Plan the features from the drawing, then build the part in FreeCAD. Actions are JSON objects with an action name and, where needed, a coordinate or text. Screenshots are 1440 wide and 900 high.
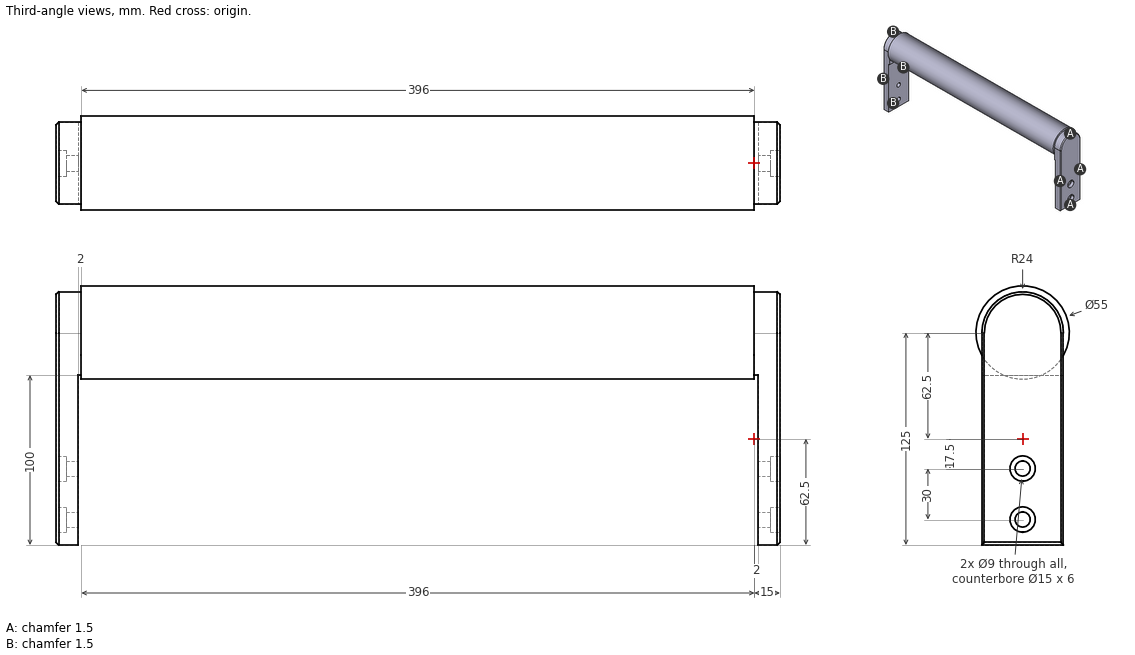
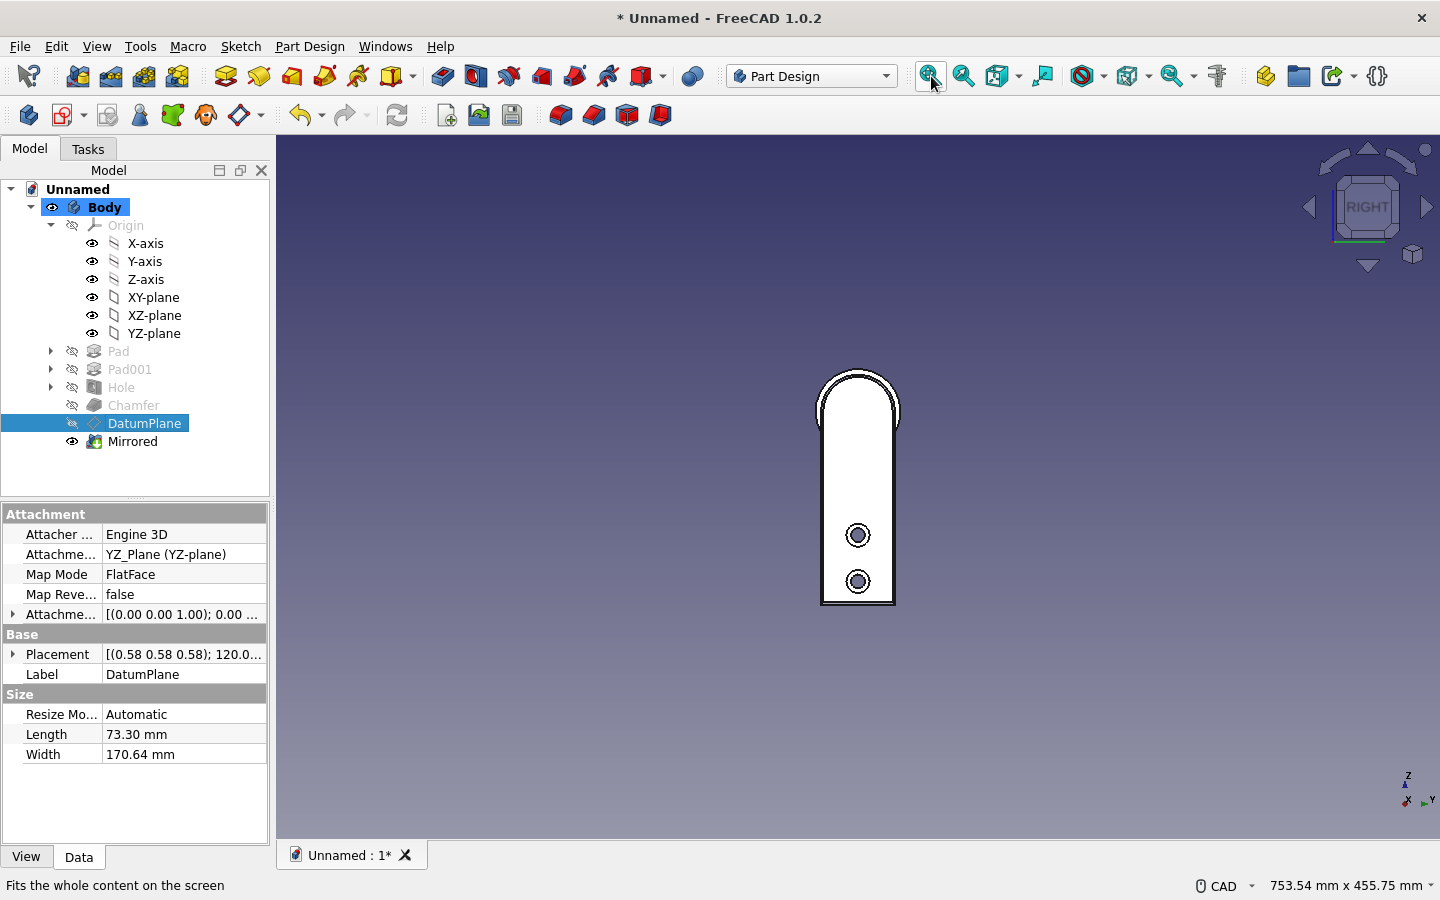
{"action": "key", "text": "0"}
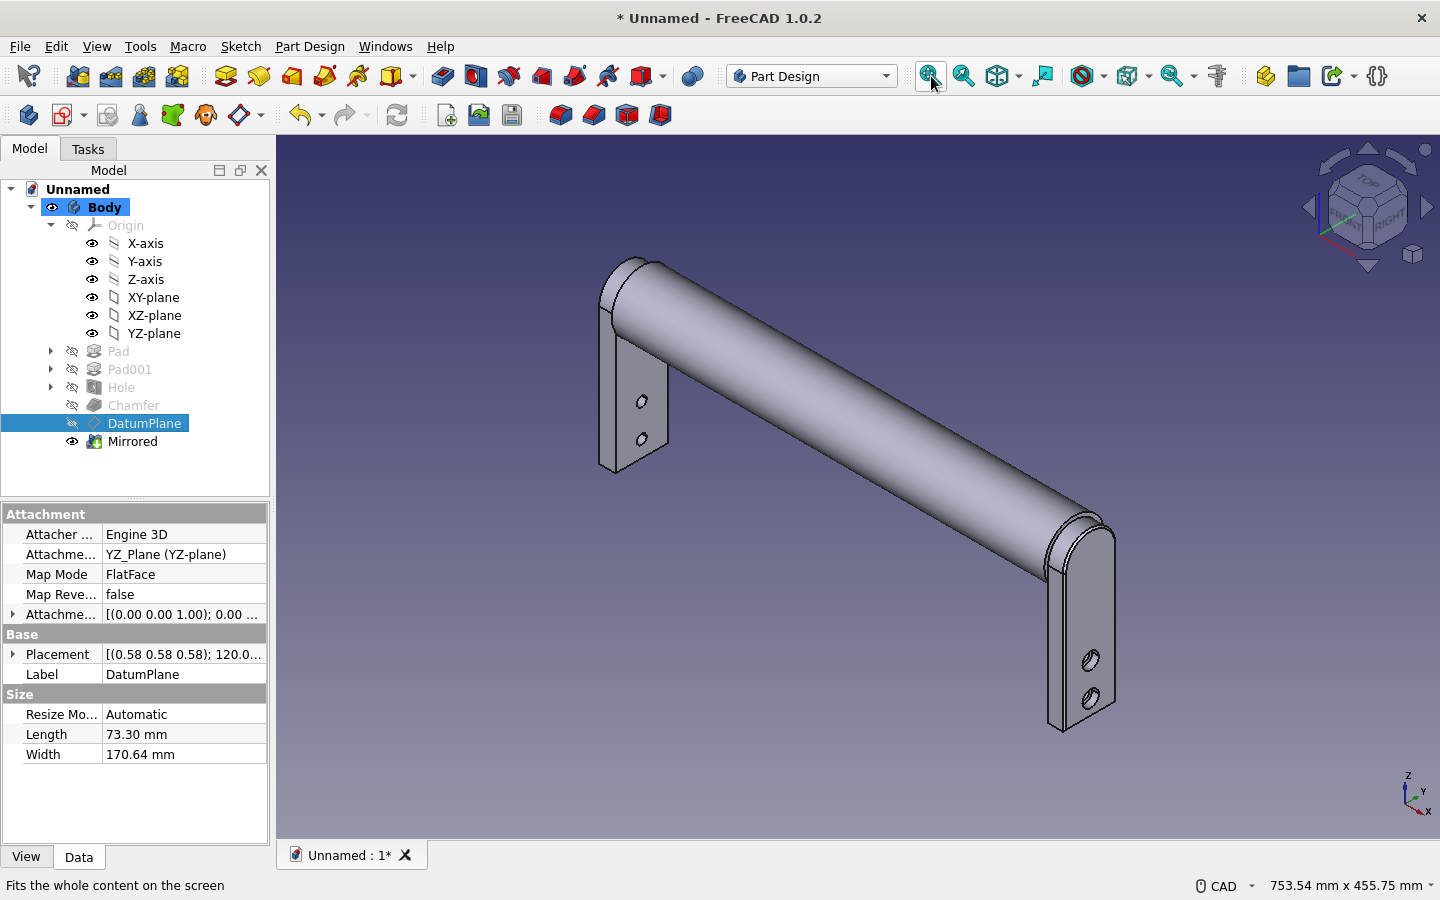
{"action": "left_click", "coordinate": [625, 260]}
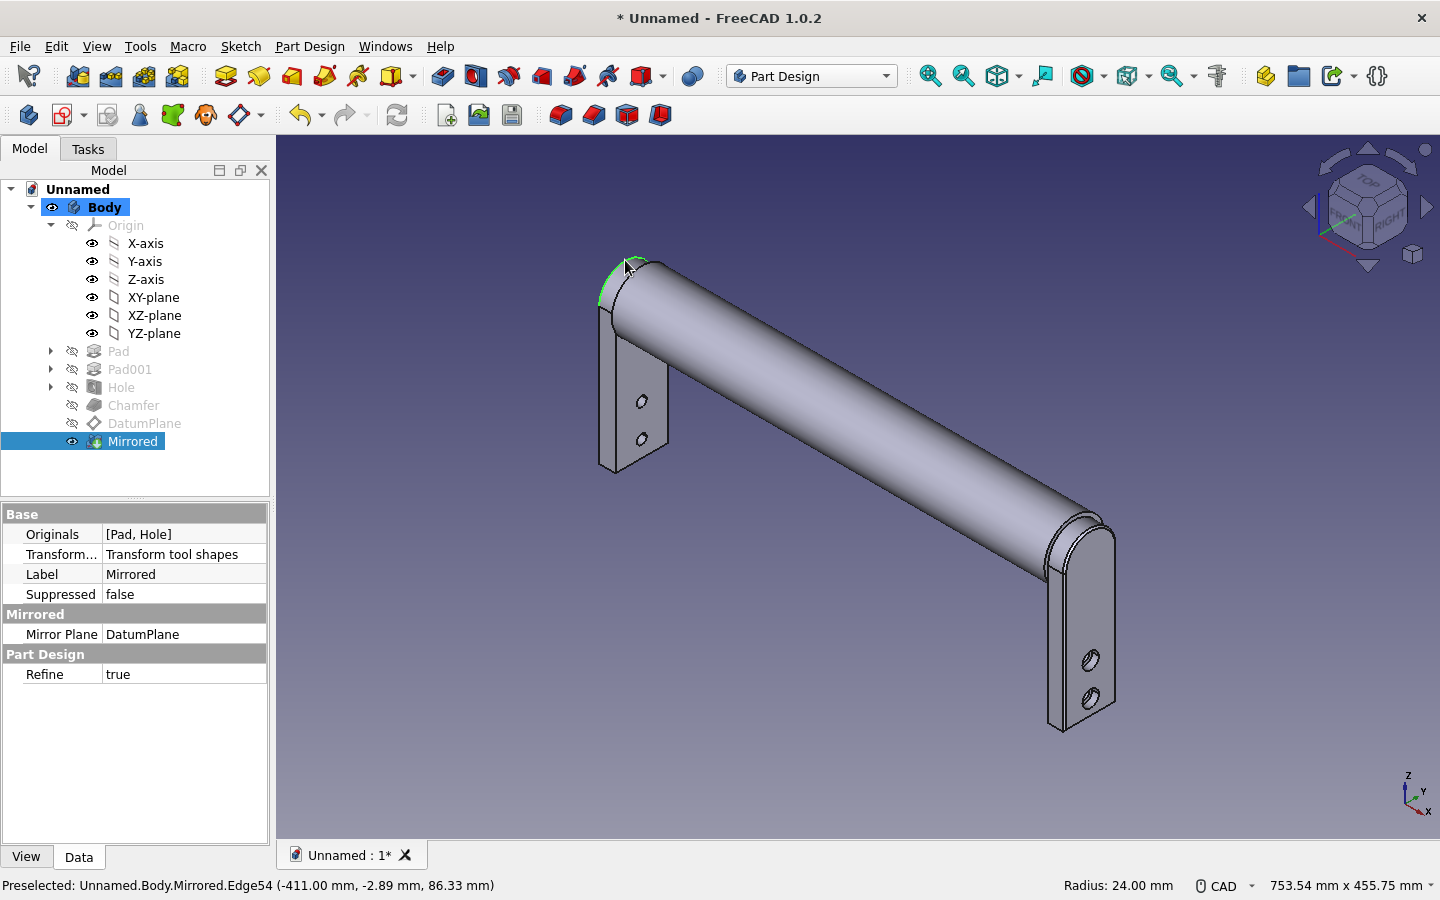
{"action": "key", "text": "2"}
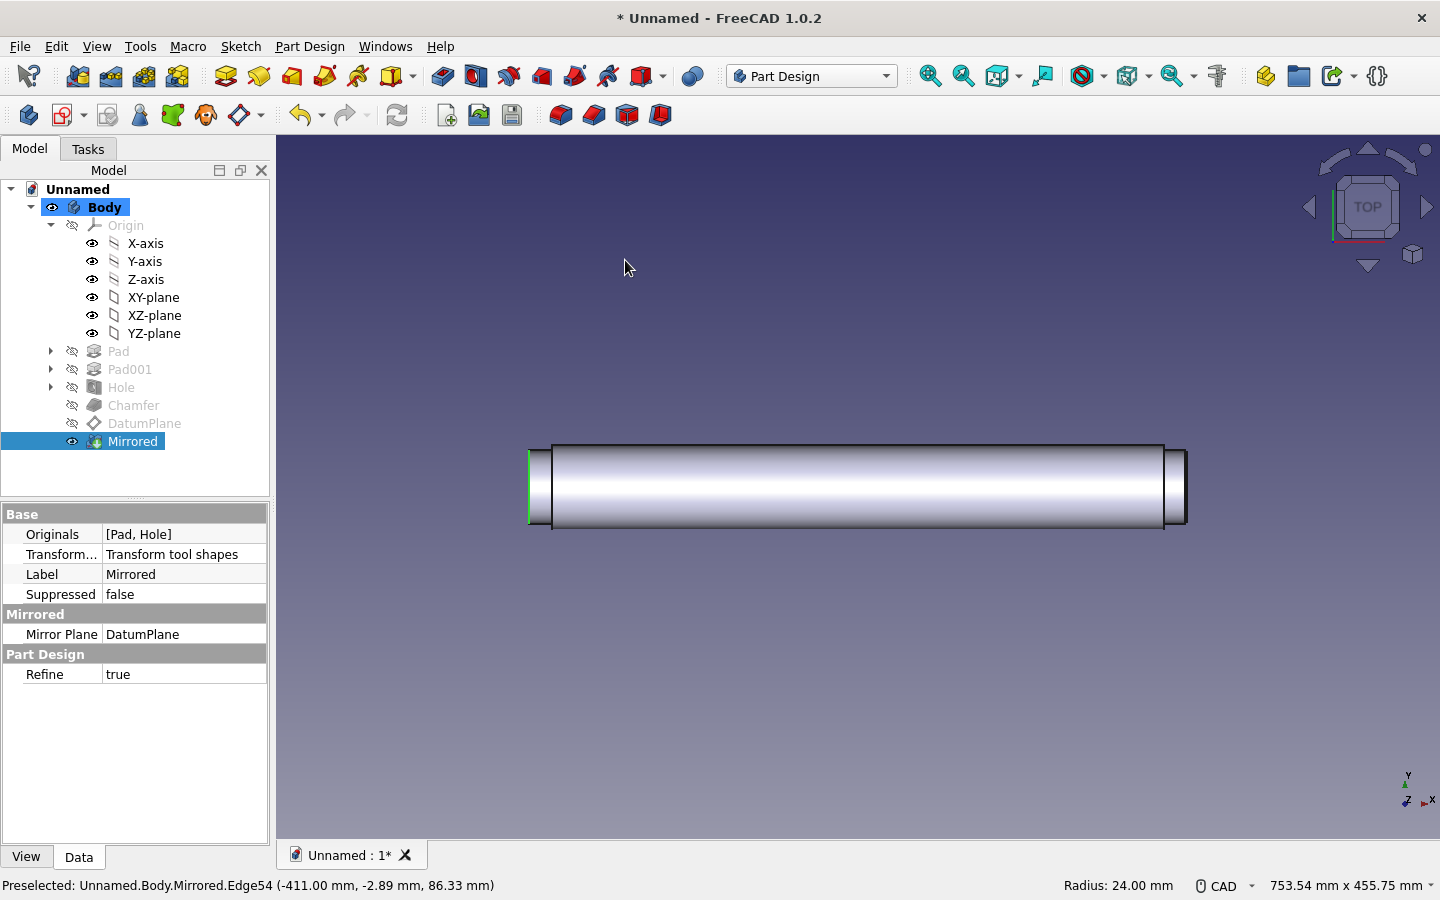
{"action": "key", "text": "1"}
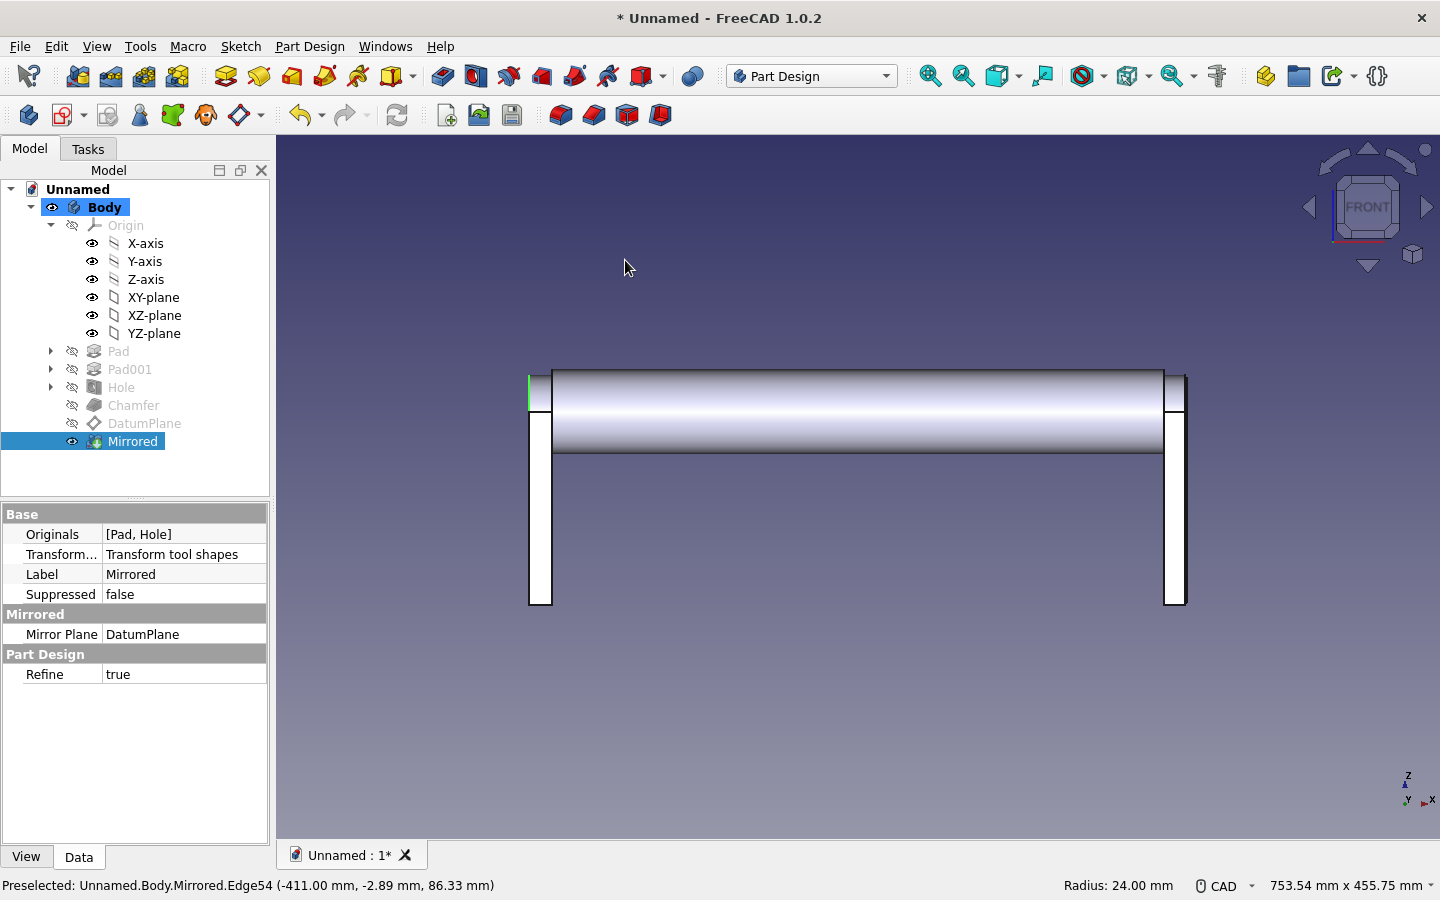
{"action": "left_click", "coordinate": [529, 507], "text": "ctrl"}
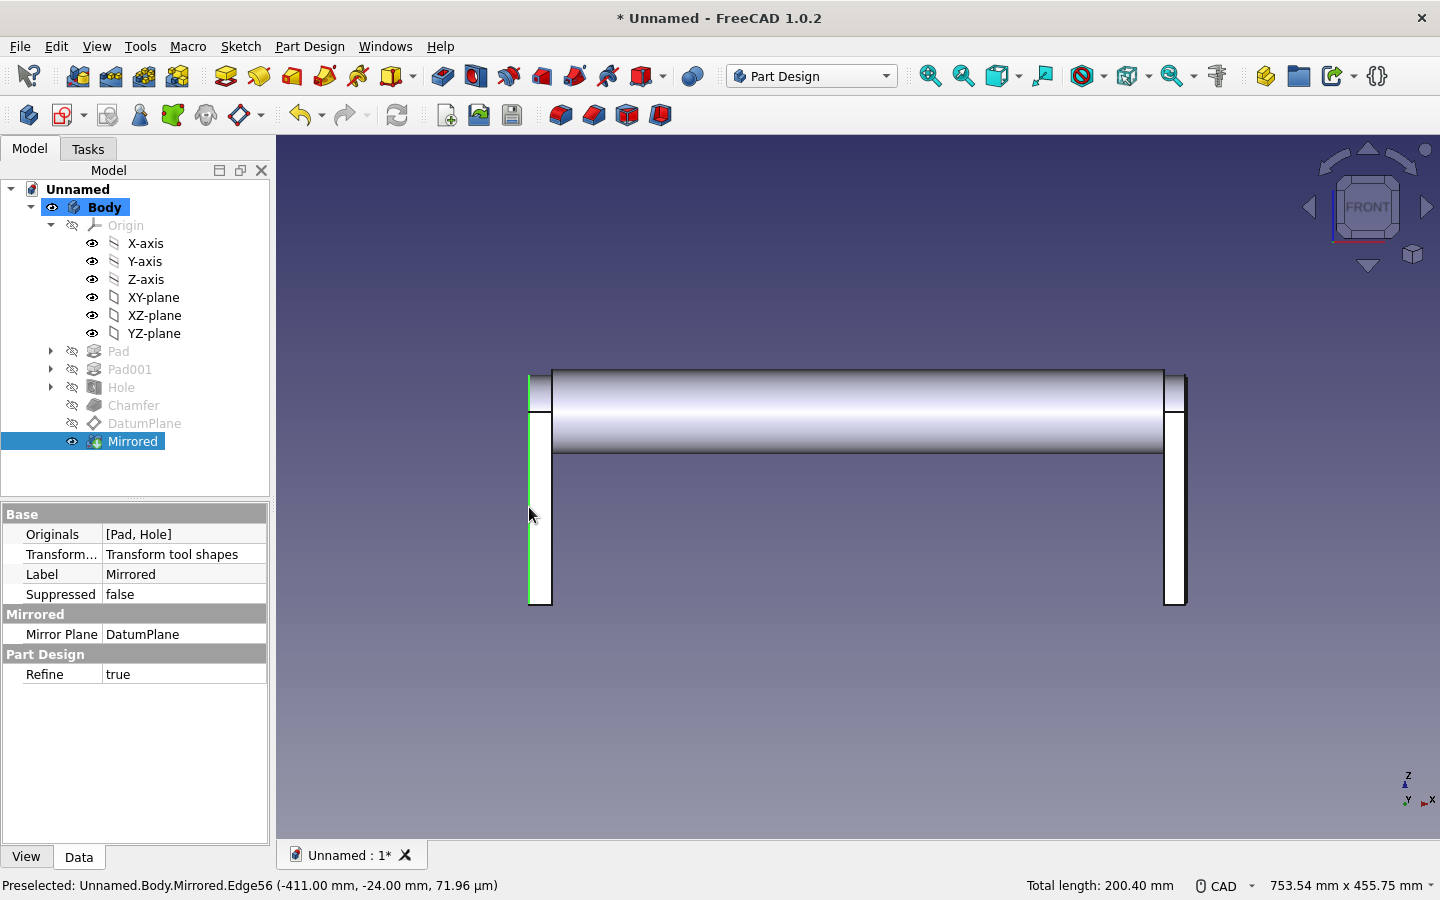
{"action": "key", "text": "3"}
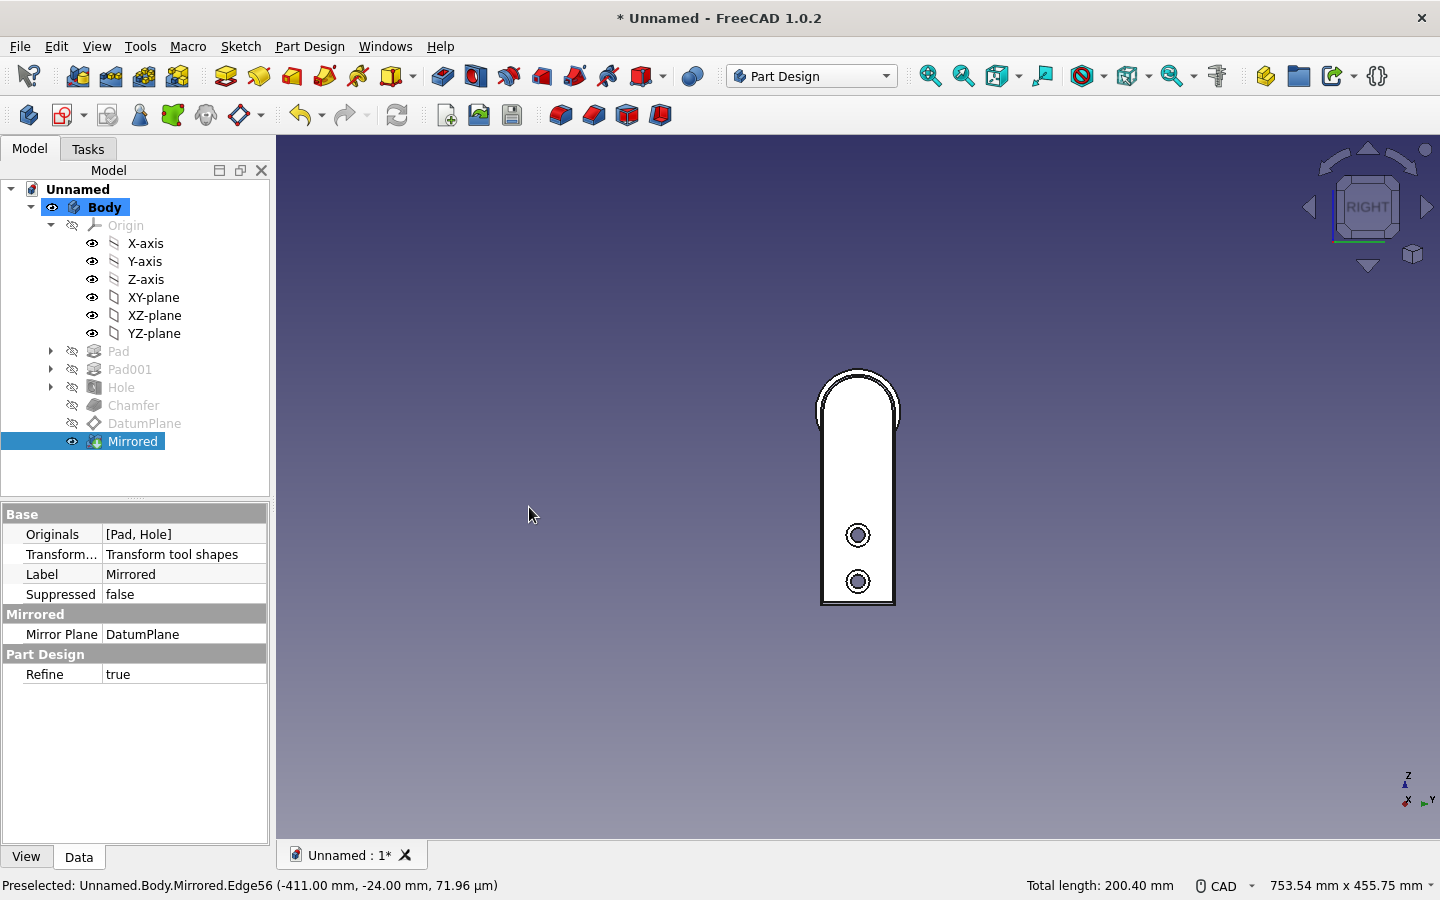
{"action": "left_click", "coordinate": [931, 76]}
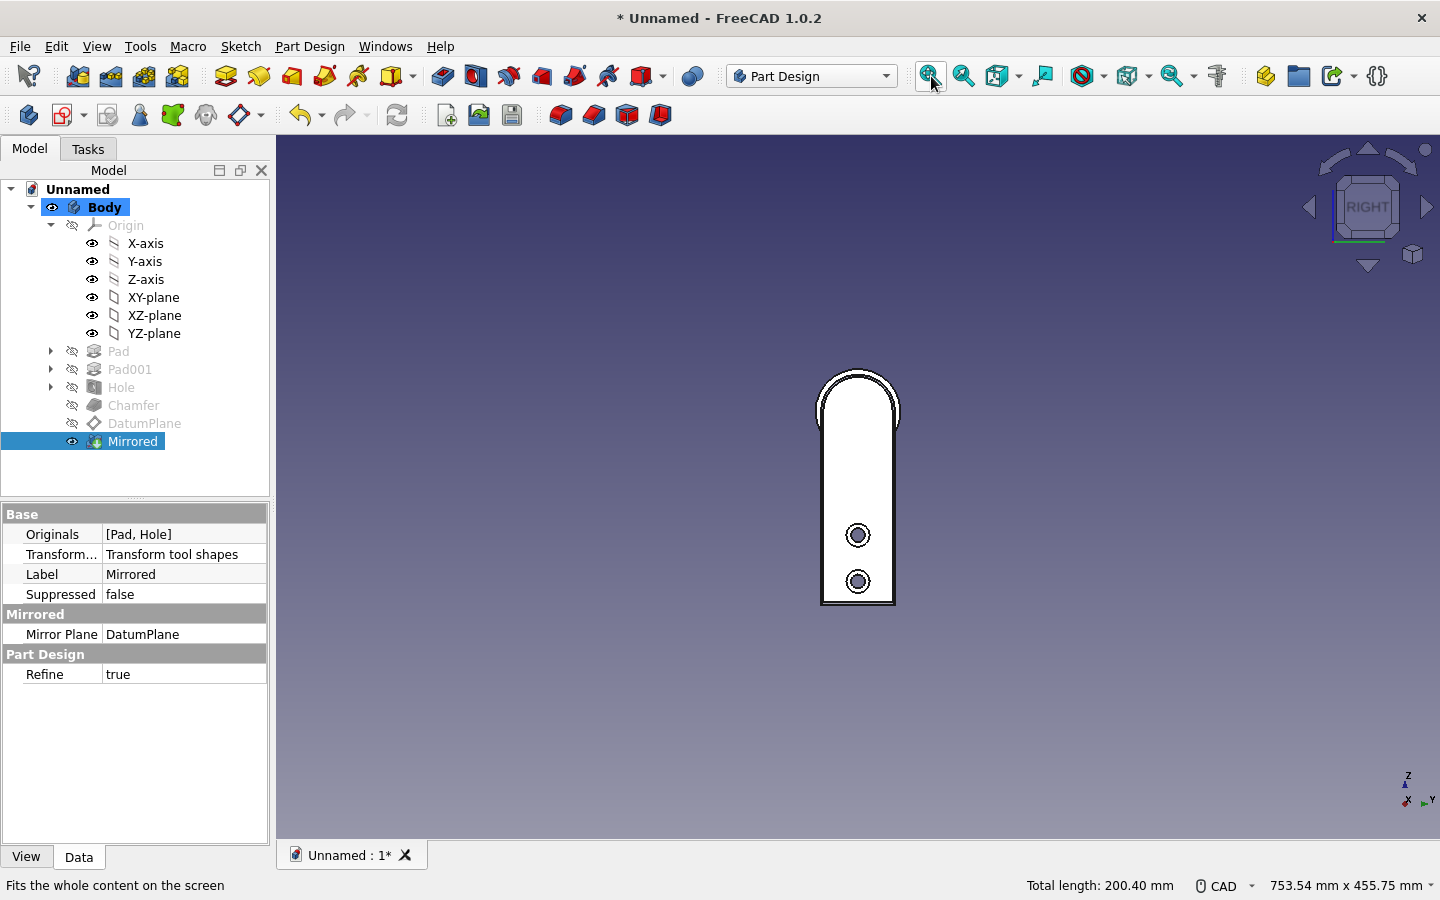
{"action": "key", "text": "5"}